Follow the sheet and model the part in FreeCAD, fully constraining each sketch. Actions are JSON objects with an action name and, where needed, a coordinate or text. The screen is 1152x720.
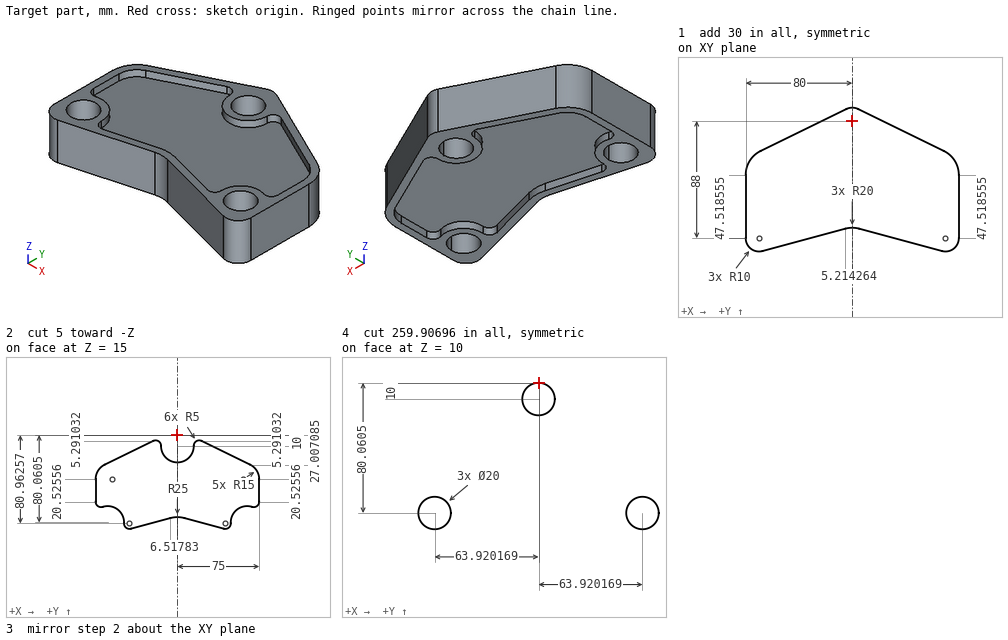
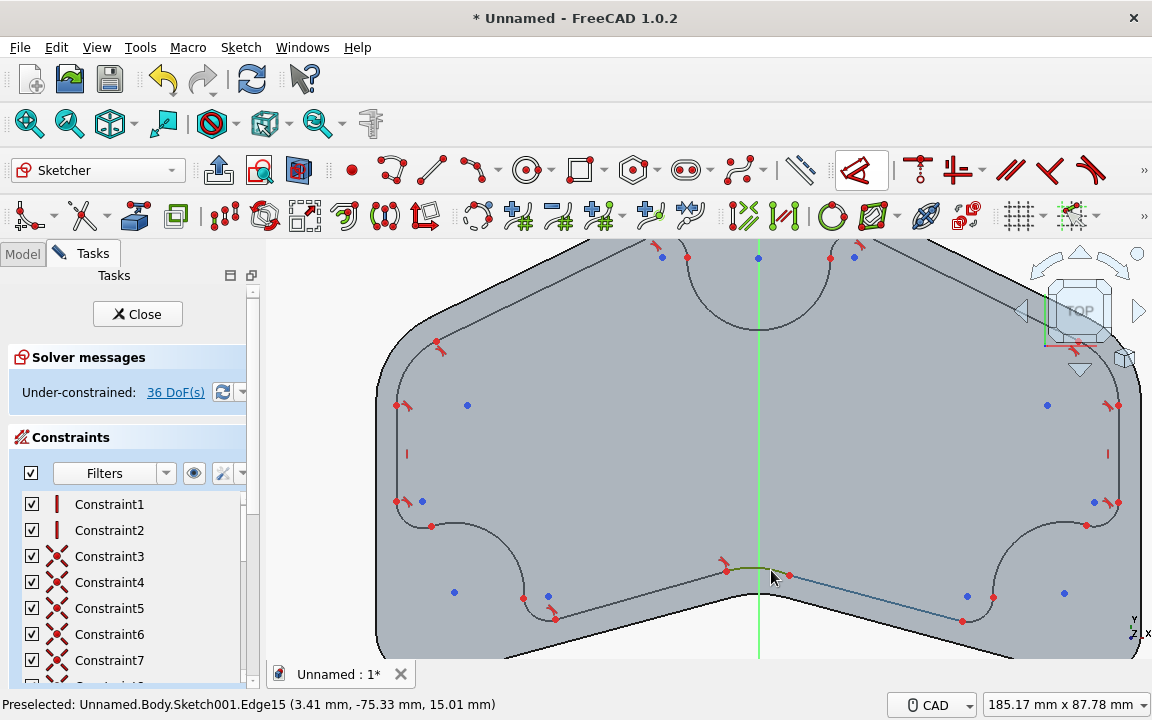
{"action": "left_click", "coordinate": [1092, 170]}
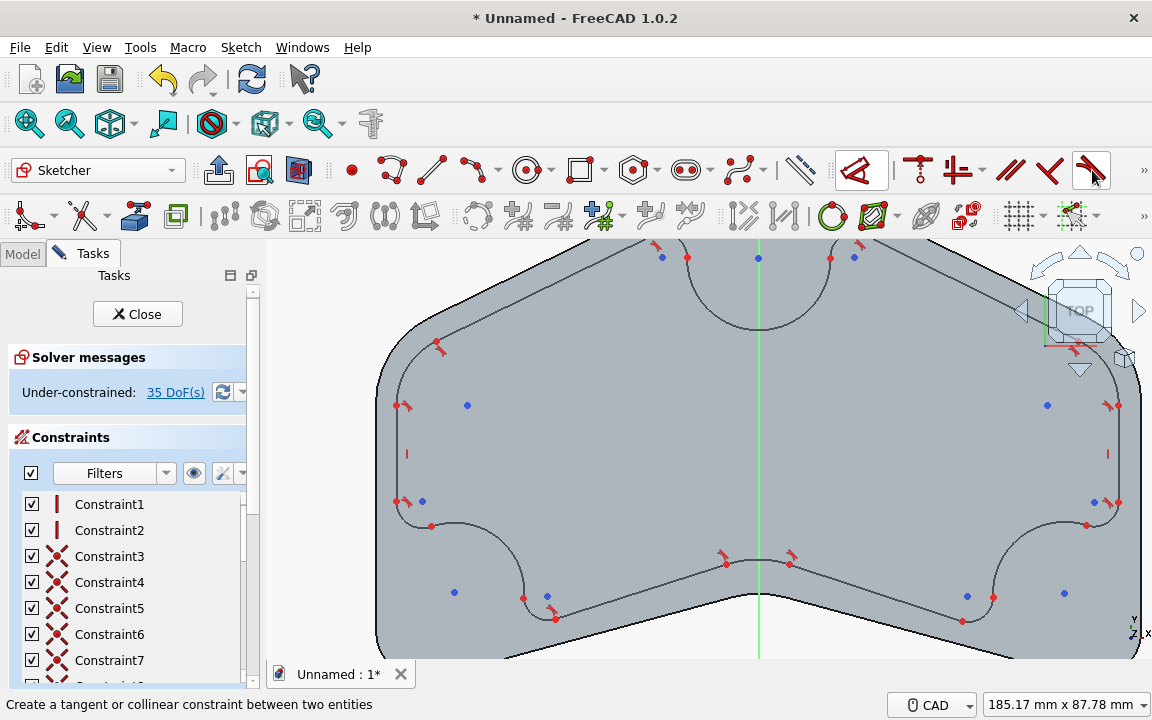
{"action": "left_click", "coordinate": [841, 582]}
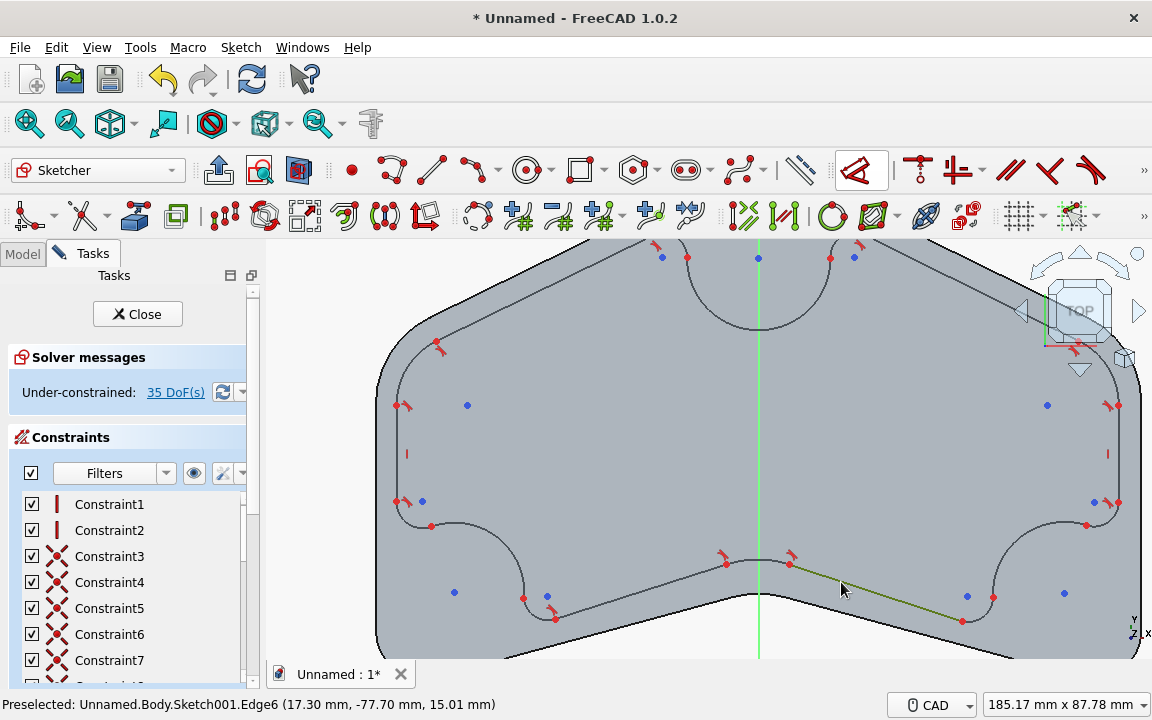
{"action": "left_click", "coordinate": [976, 621]}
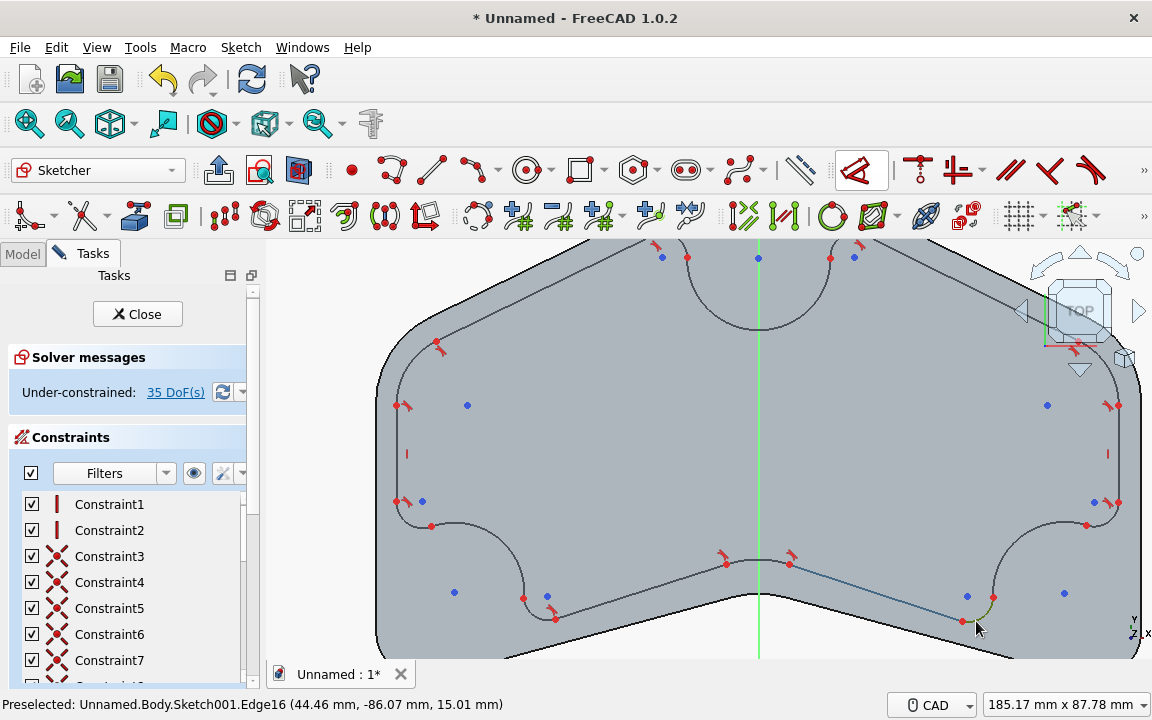
{"action": "left_click", "coordinate": [1092, 170]}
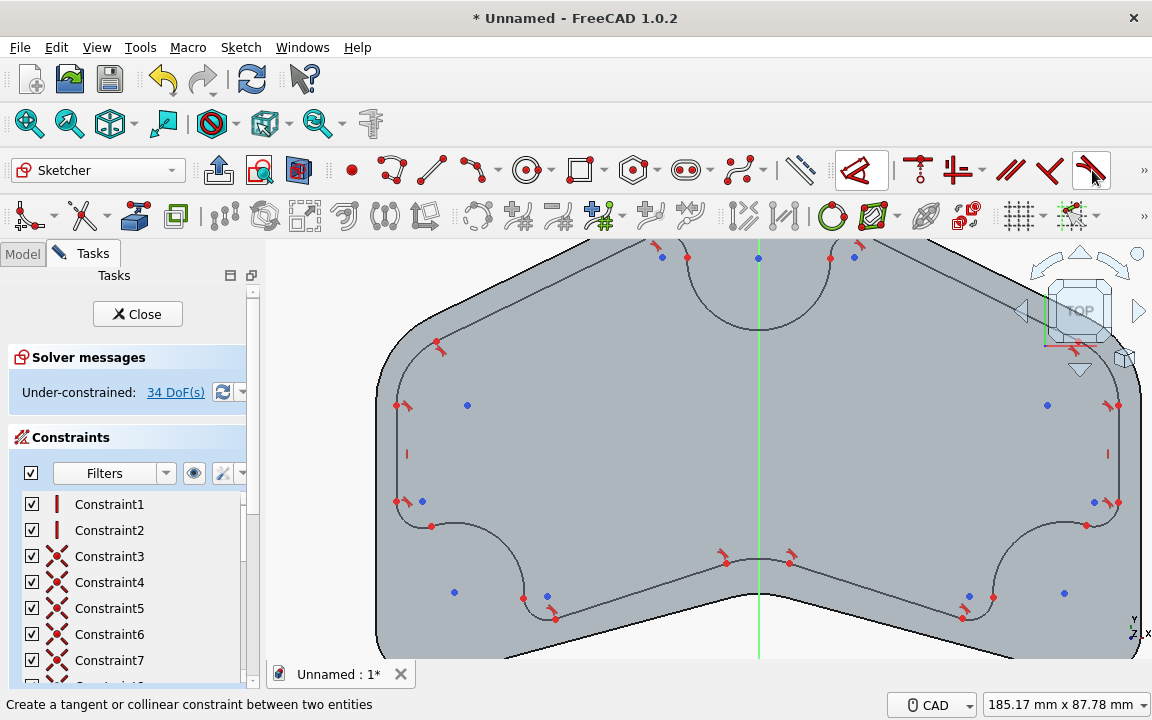
{"action": "scroll", "coordinate": [400, 518], "scroll_direction": "down", "scroll_amount": 2}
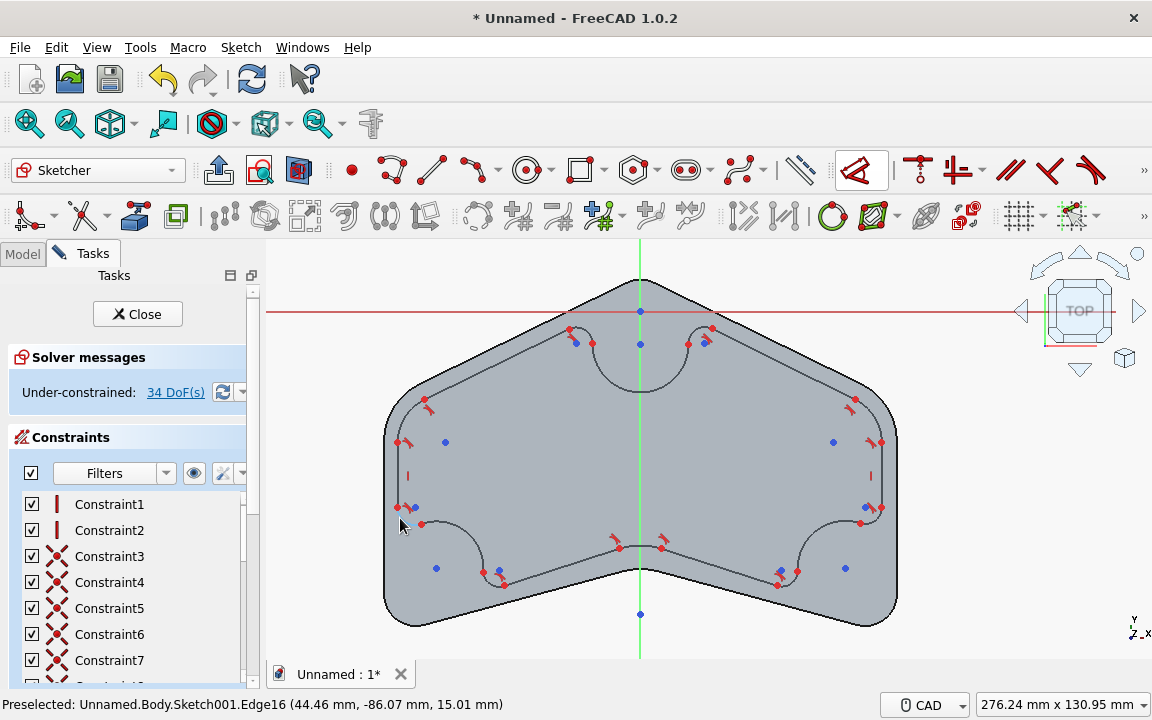
{"action": "scroll", "coordinate": [702, 327], "scroll_direction": "up", "scroll_amount": 2}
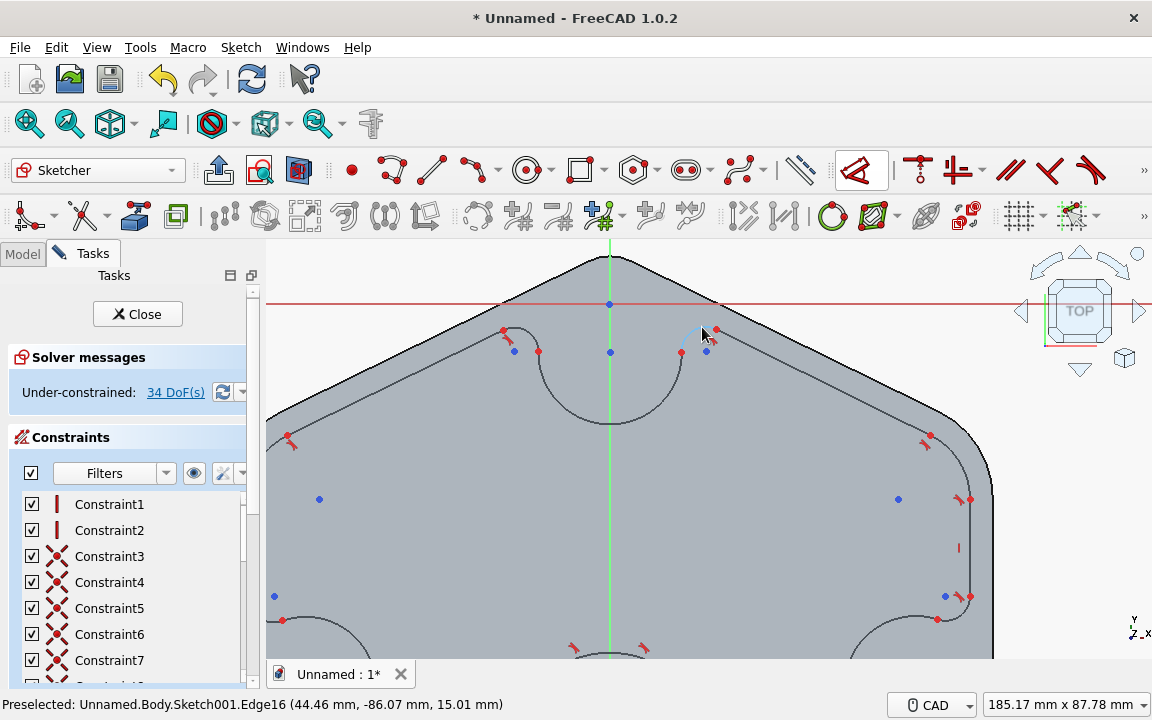
{"action": "left_click", "coordinate": [702, 327]}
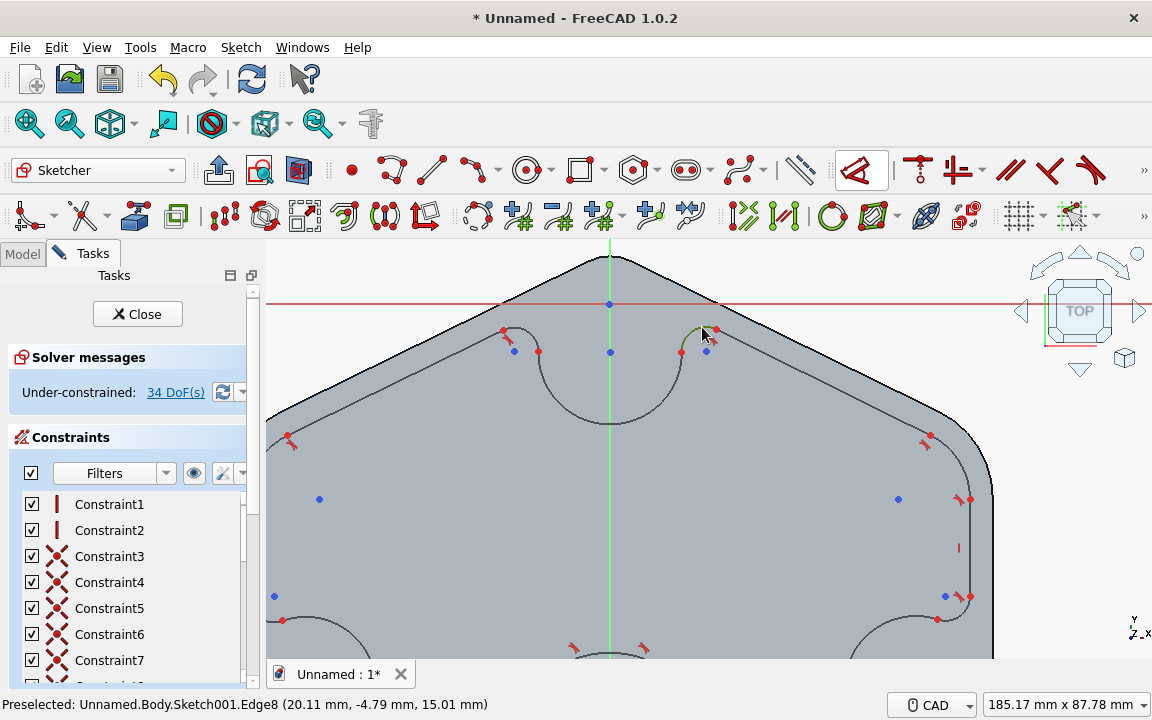
{"action": "left_click", "coordinate": [567, 410]}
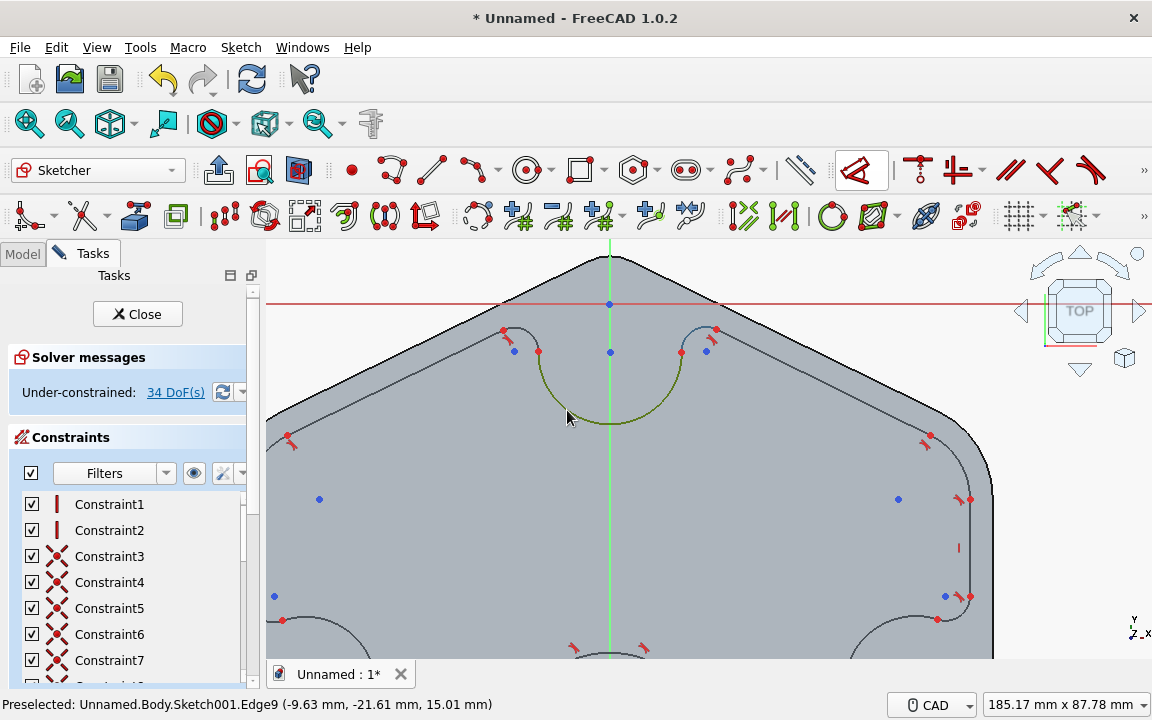
{"action": "key", "text": "t"}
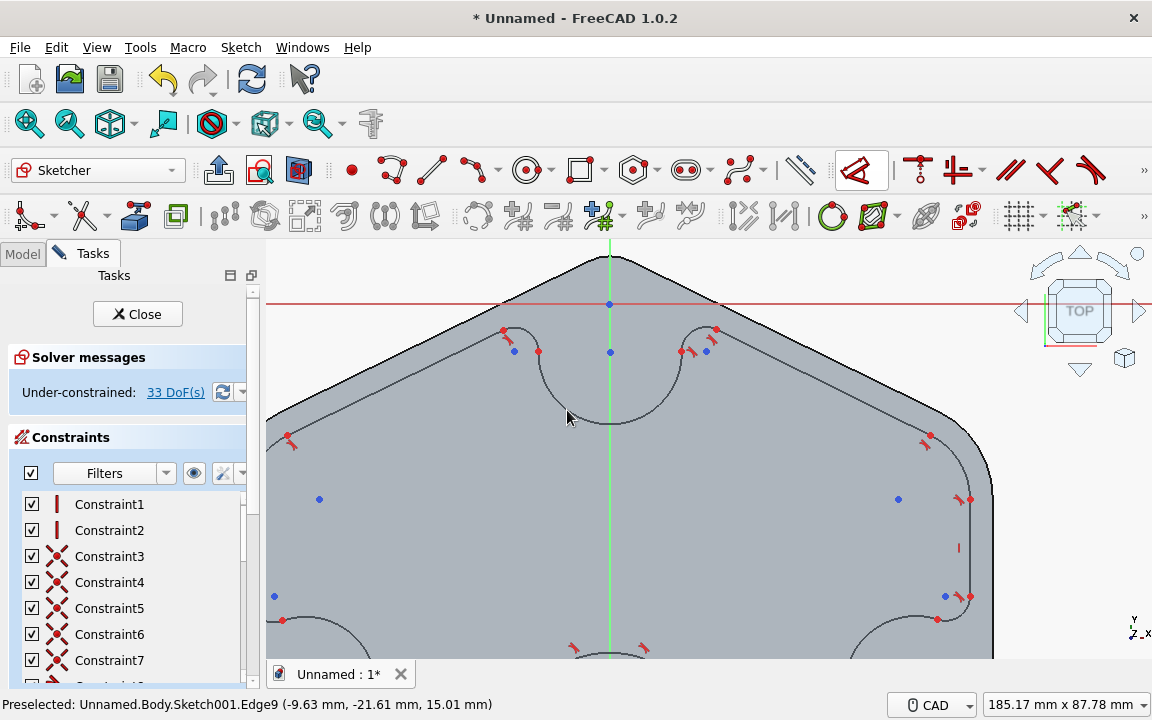
{"action": "left_click", "coordinate": [568, 410]}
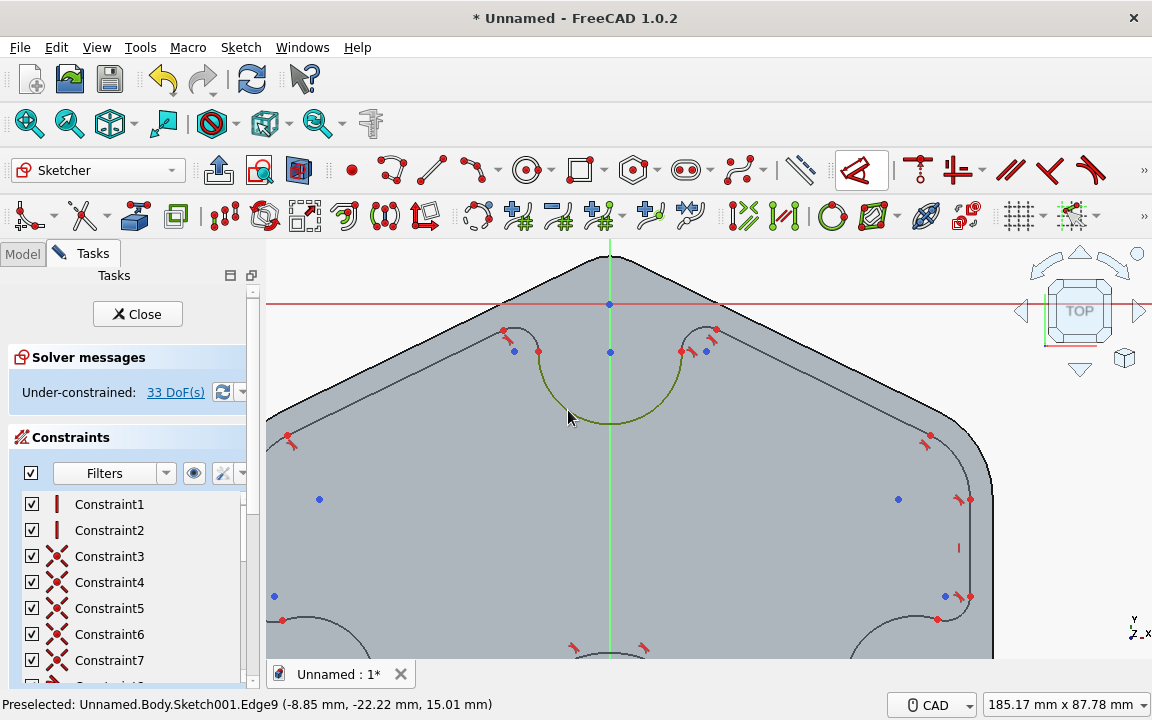
{"action": "left_click", "coordinate": [534, 338]}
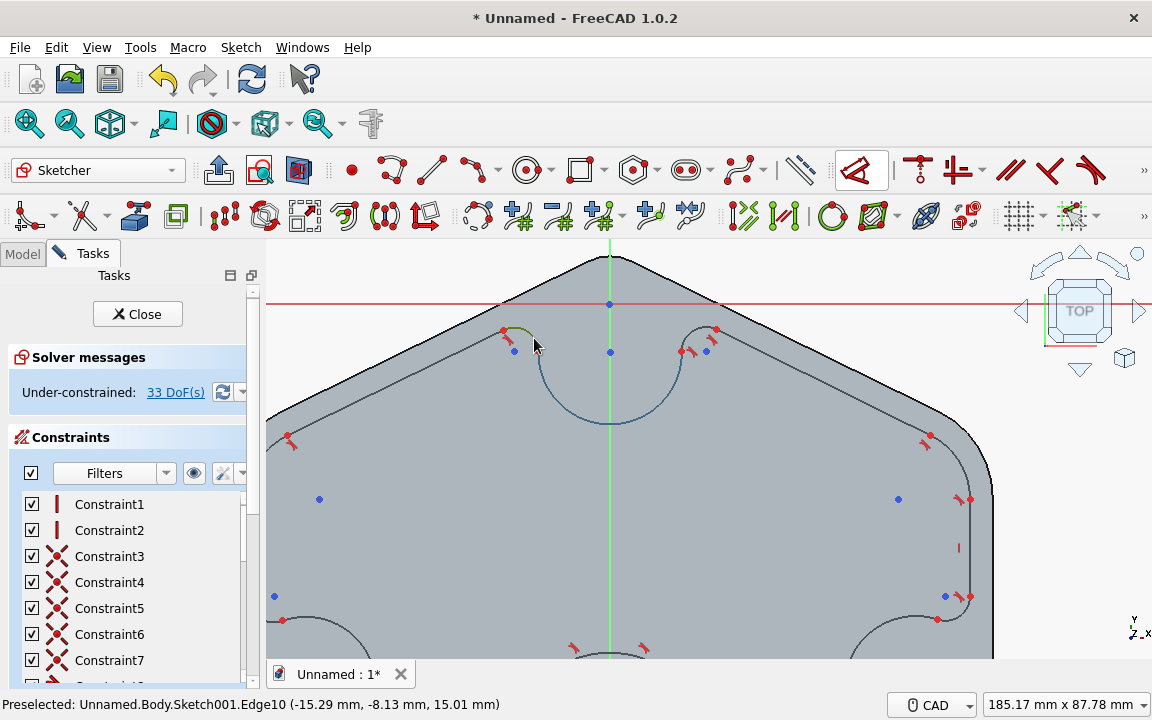
{"action": "left_click", "coordinate": [1092, 170]}